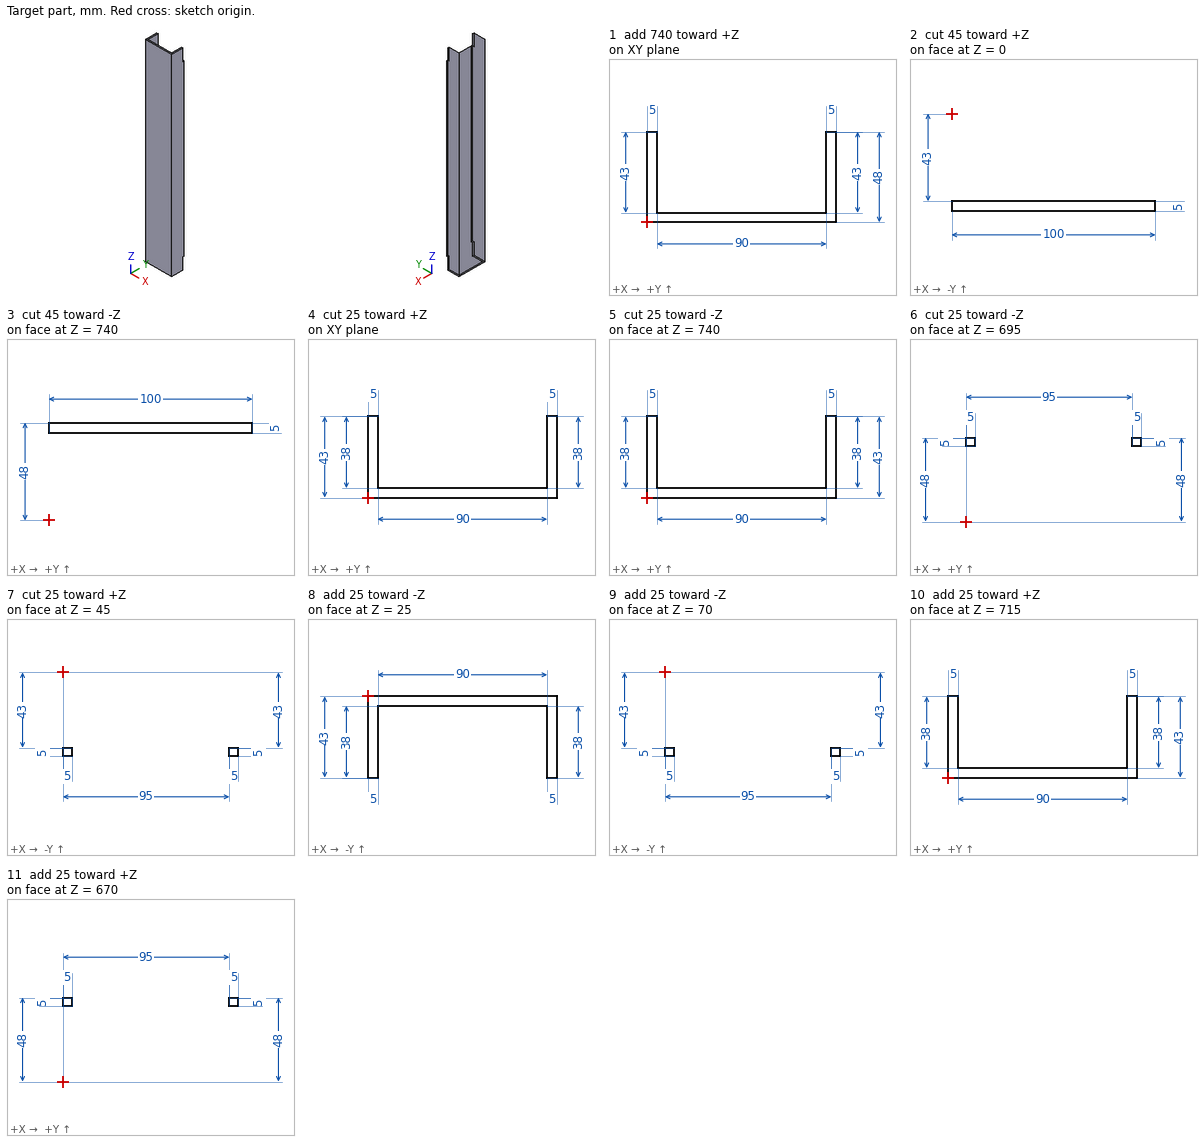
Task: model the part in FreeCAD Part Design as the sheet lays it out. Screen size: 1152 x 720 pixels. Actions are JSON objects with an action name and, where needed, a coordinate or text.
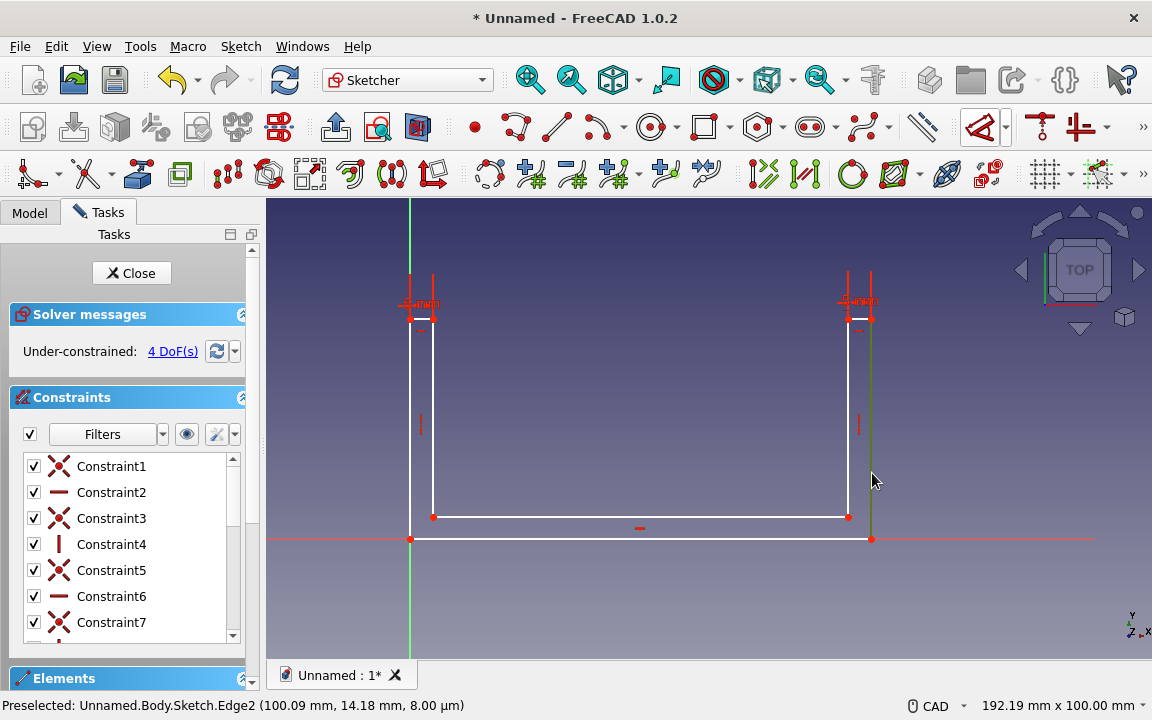
{"action": "key", "text": "i"}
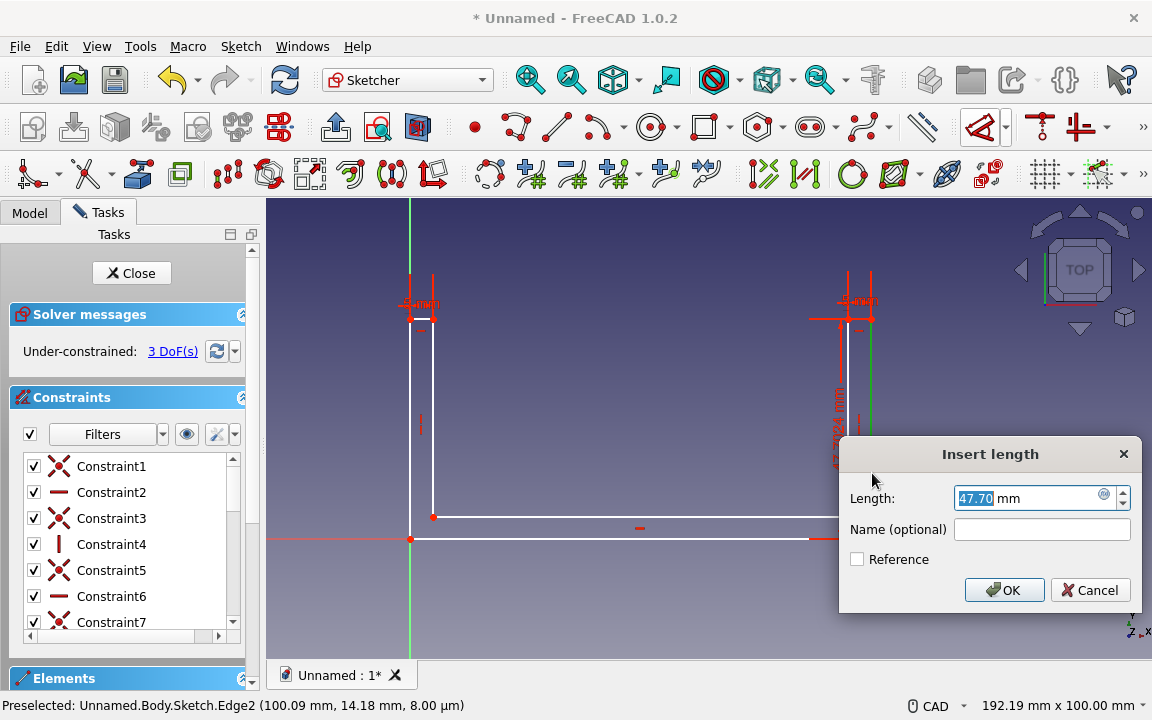
{"action": "type", "text": "48"}
{"action": "key", "text": "Return"}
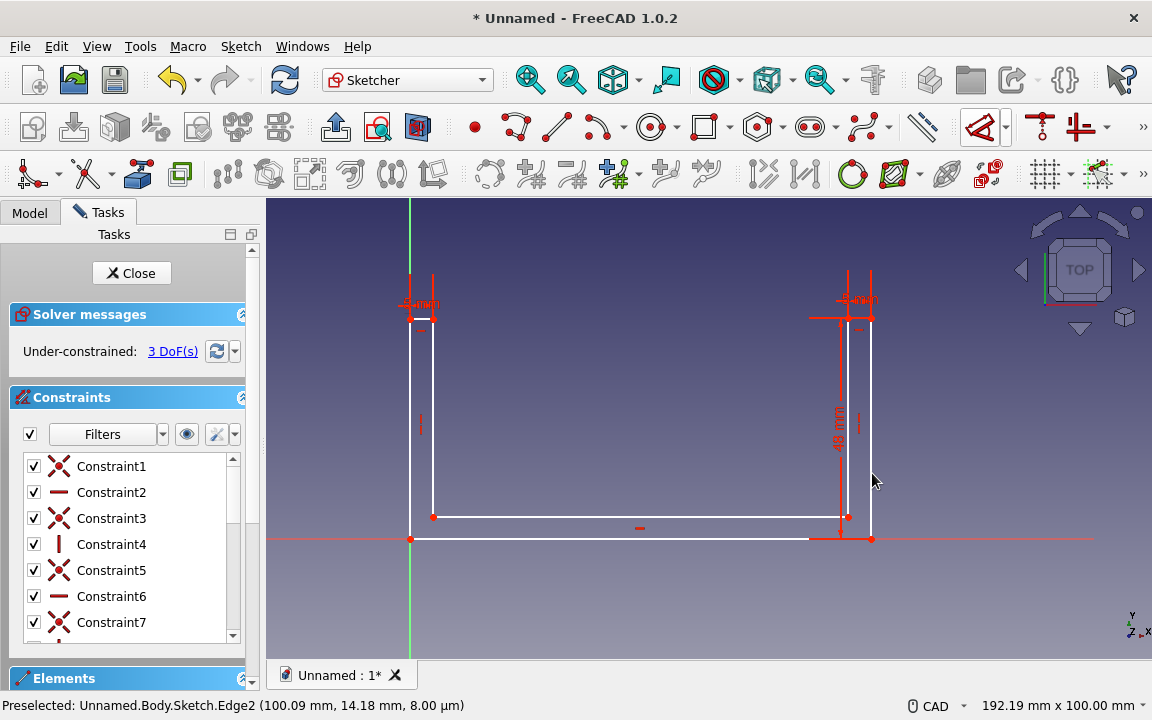
{"action": "left_click", "coordinate": [848, 378]}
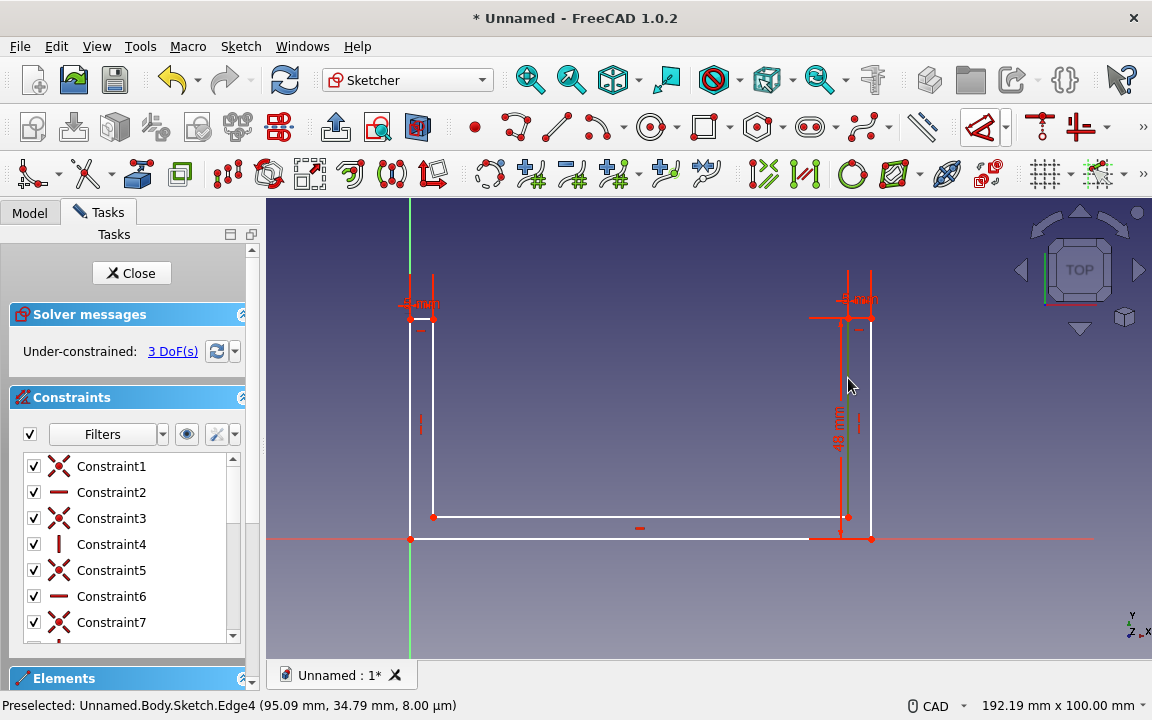
{"action": "key", "text": "i"}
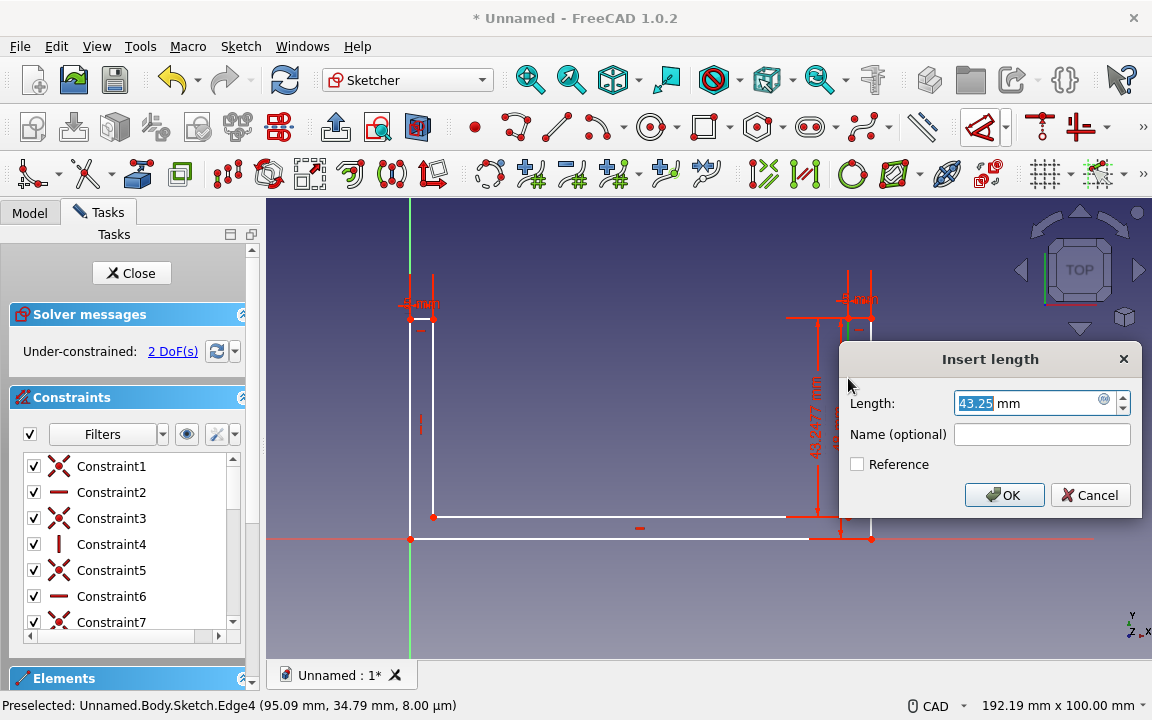
{"action": "type", "text": "43"}
{"action": "key", "text": "Return"}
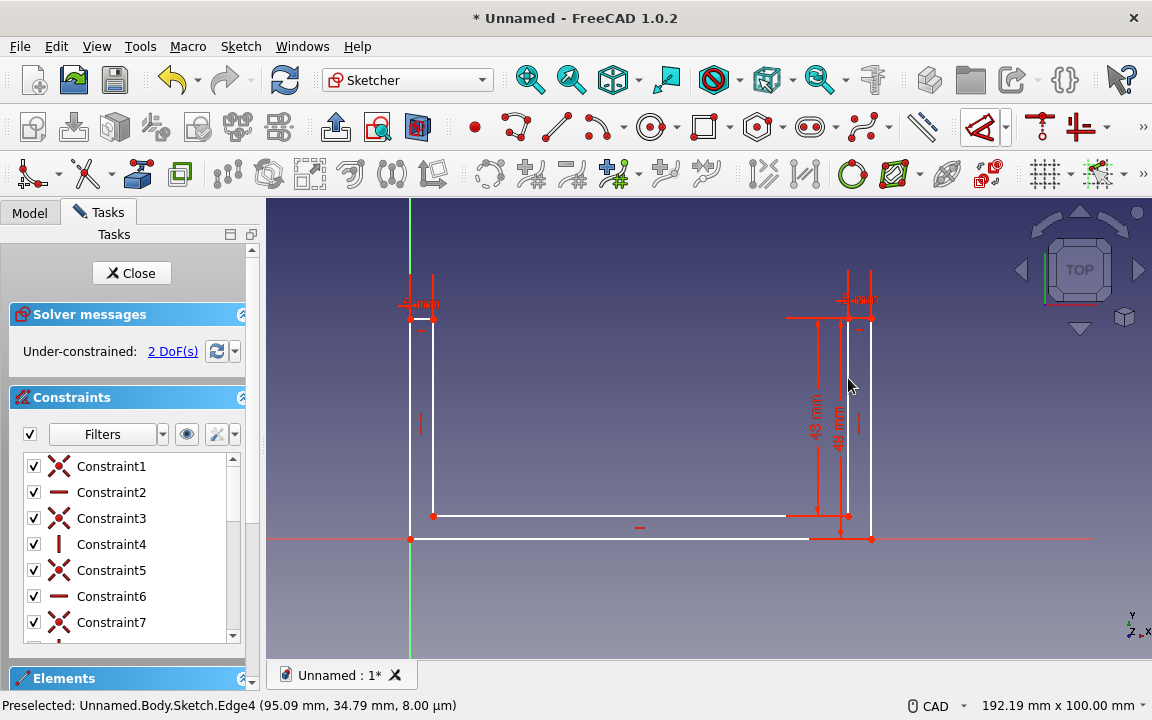
{"action": "left_click", "coordinate": [724, 516]}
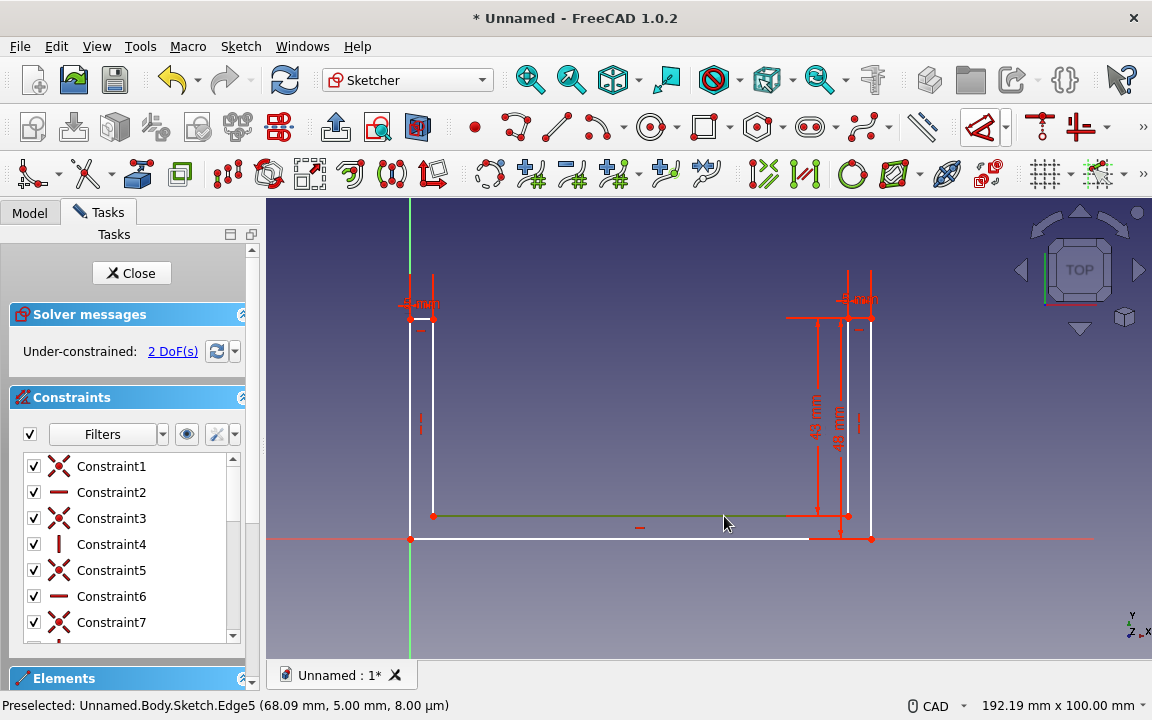
{"action": "key", "text": "l"}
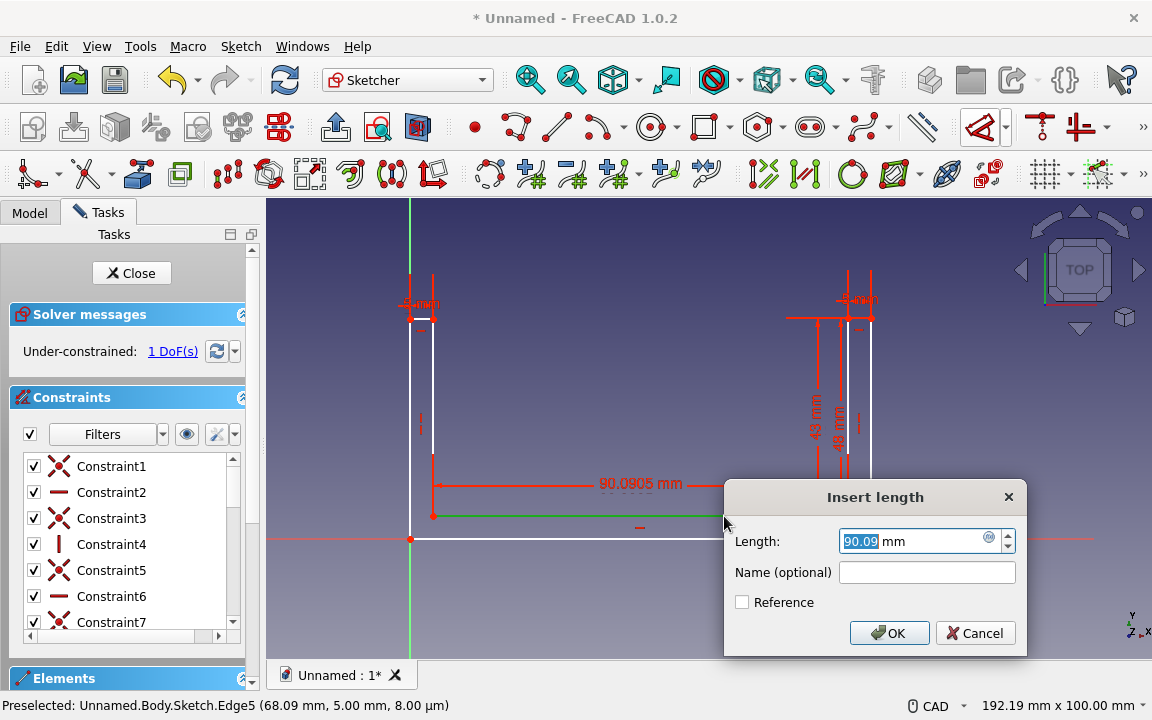
{"action": "type", "text": "90"}
{"action": "key", "text": "Return"}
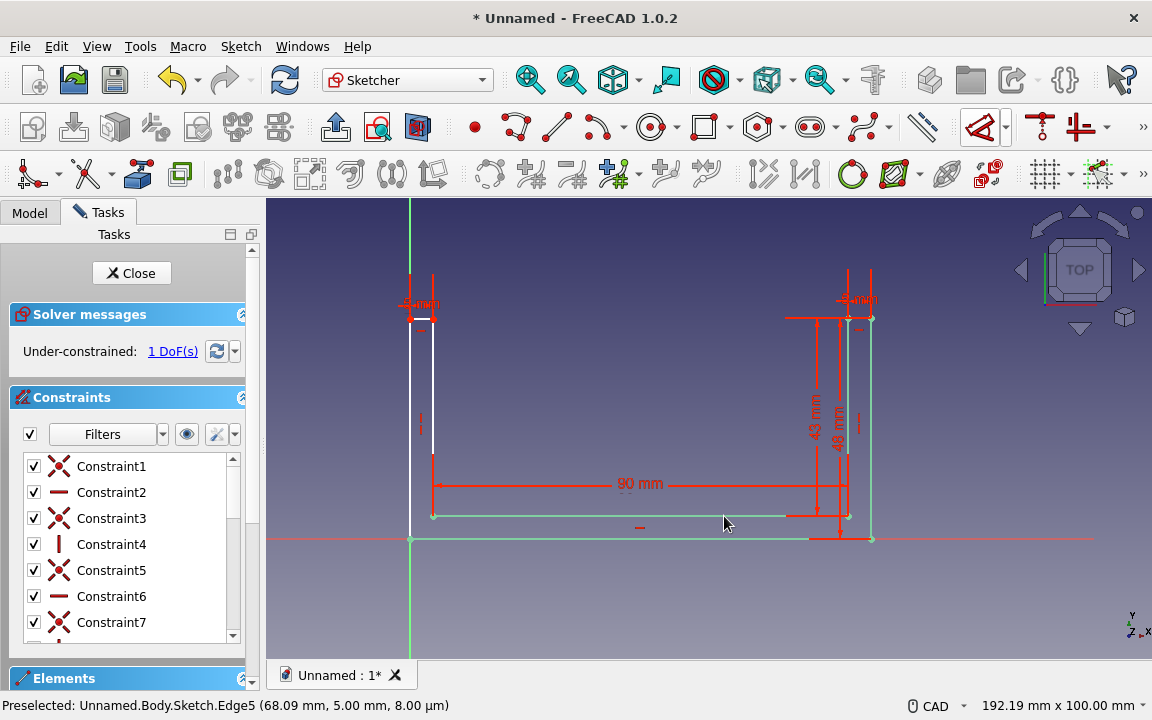
{"action": "left_click", "coordinate": [433, 457]}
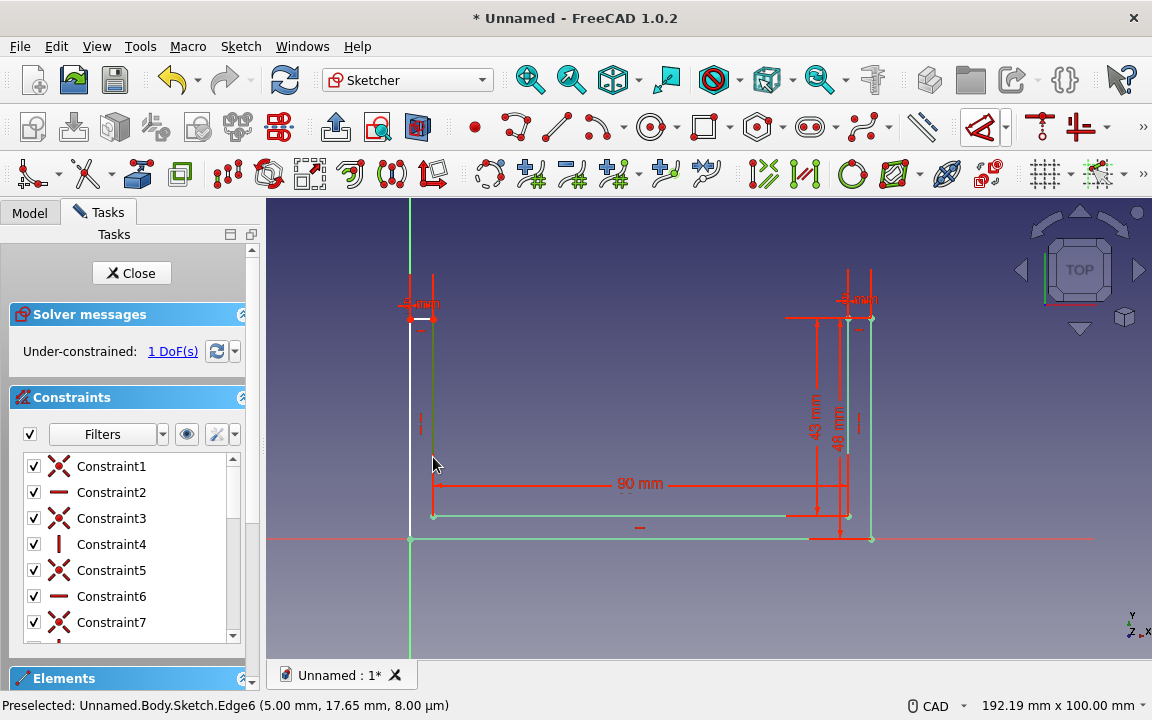
{"action": "key", "text": "i"}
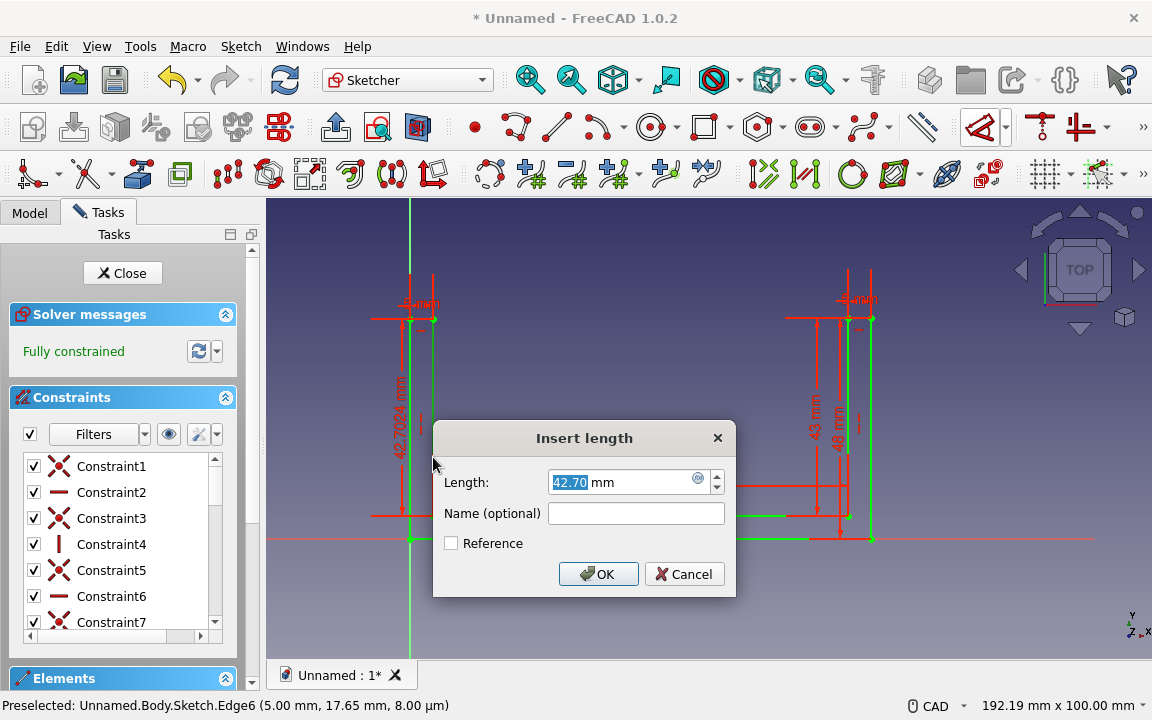
{"action": "type", "text": "43"}
{"action": "key", "text": "Return"}